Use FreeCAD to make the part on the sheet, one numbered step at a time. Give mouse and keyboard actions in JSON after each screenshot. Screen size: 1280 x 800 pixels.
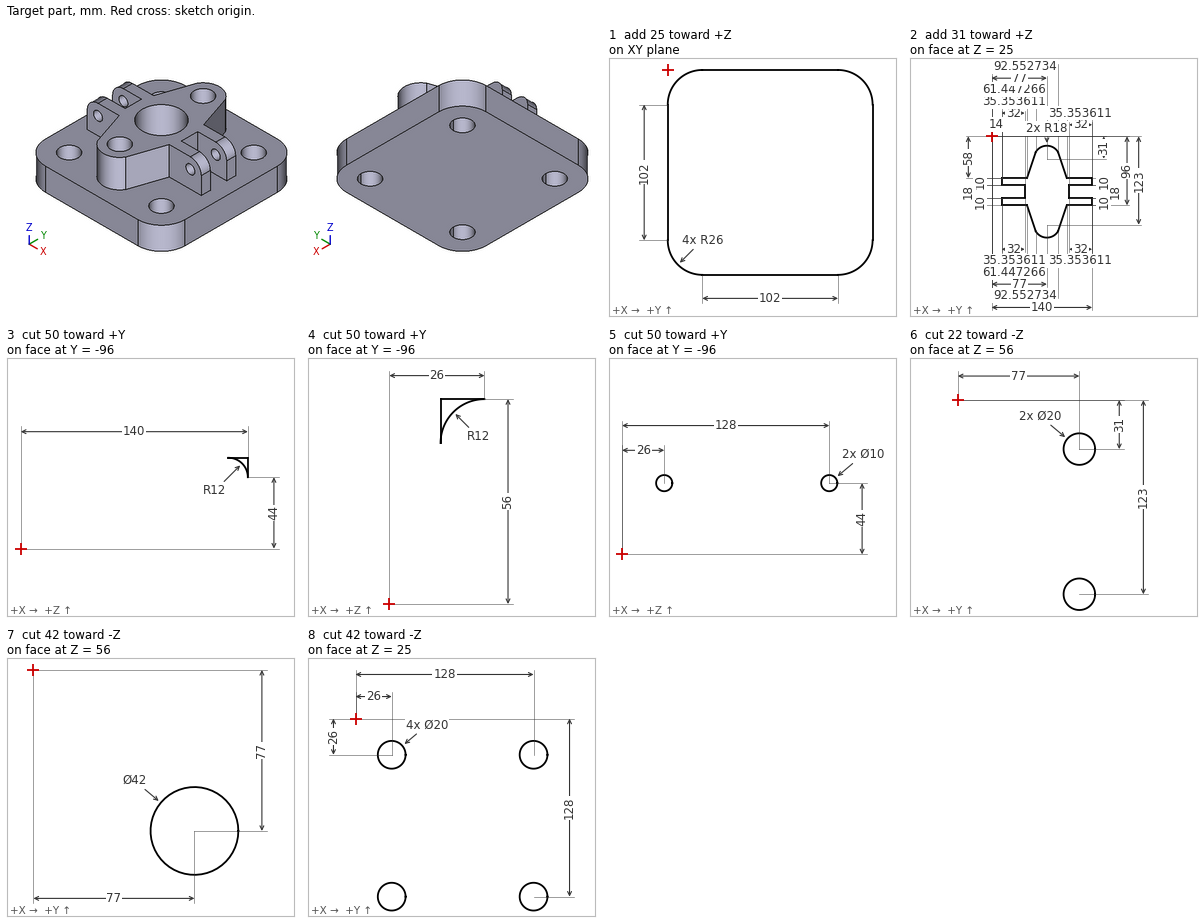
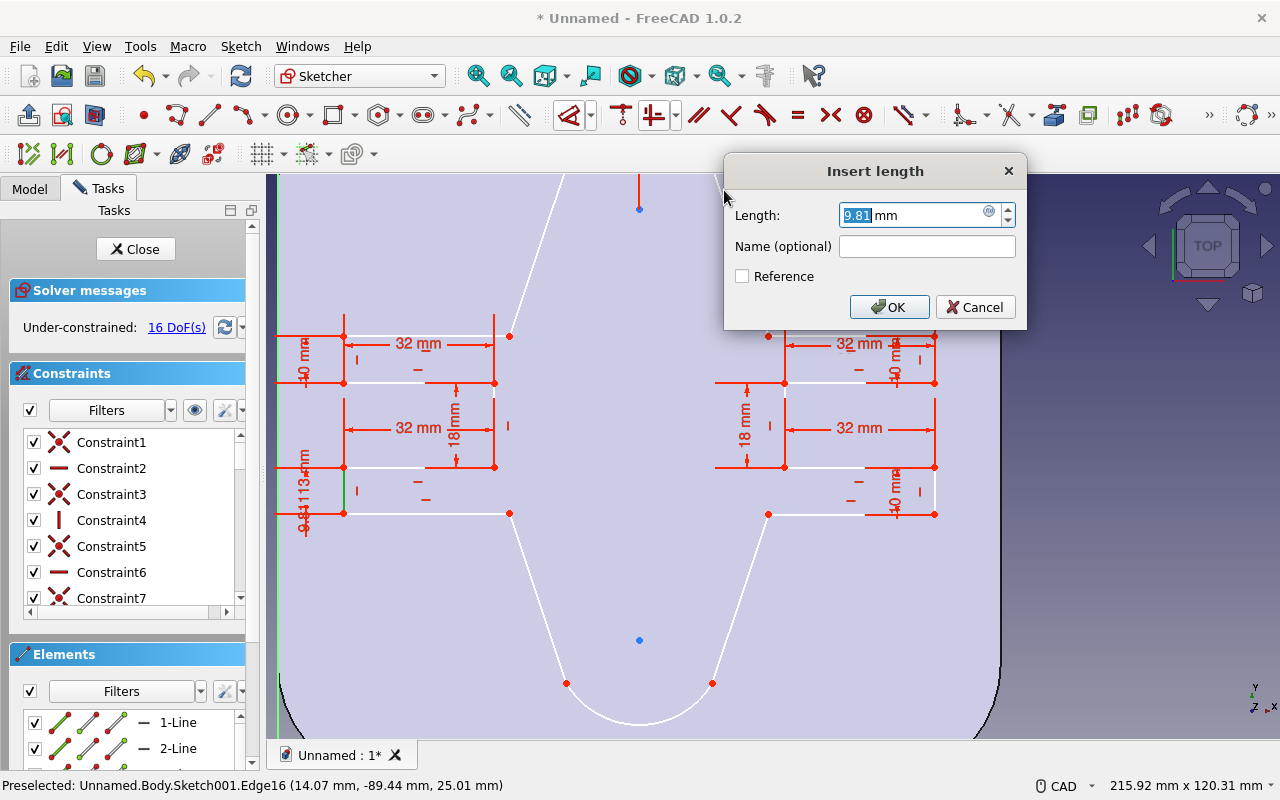
{"action": "type", "text": "10"}
{"action": "key", "text": "Return"}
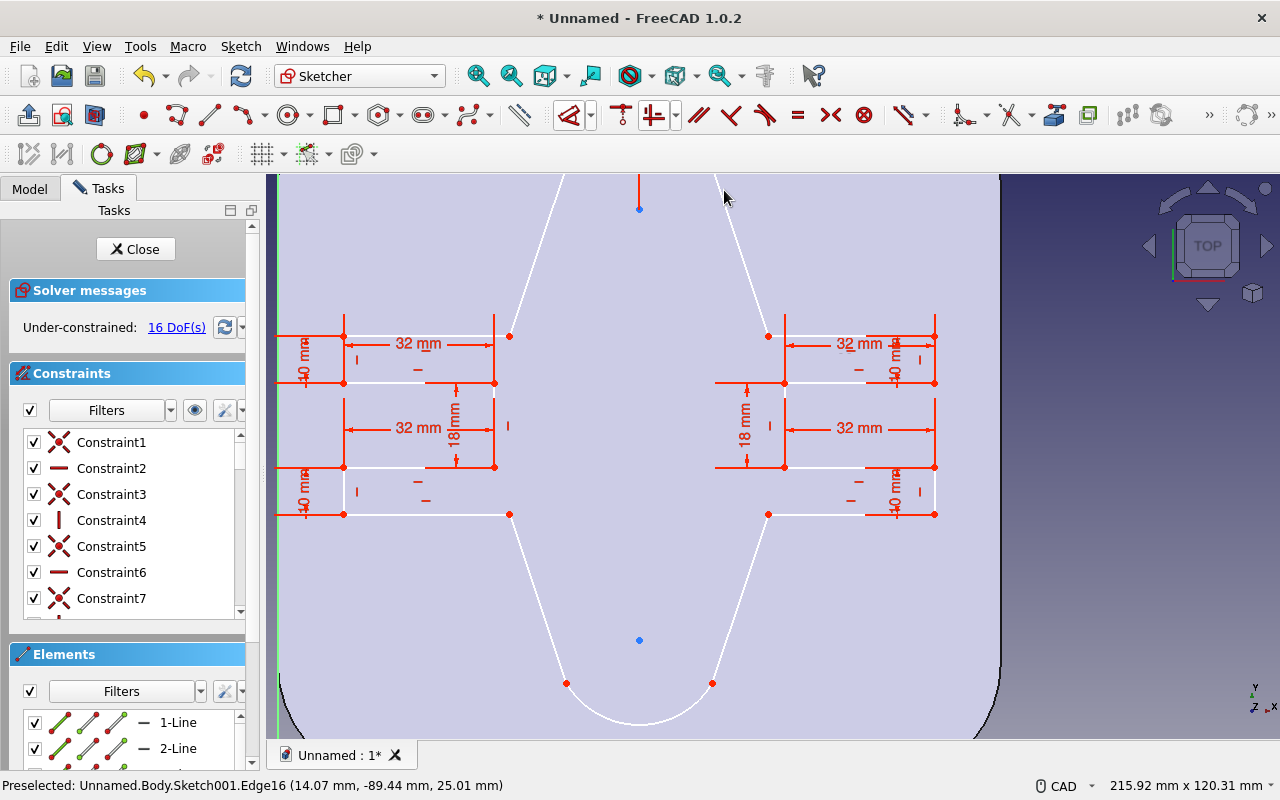
{"action": "left_click", "coordinate": [769, 515]}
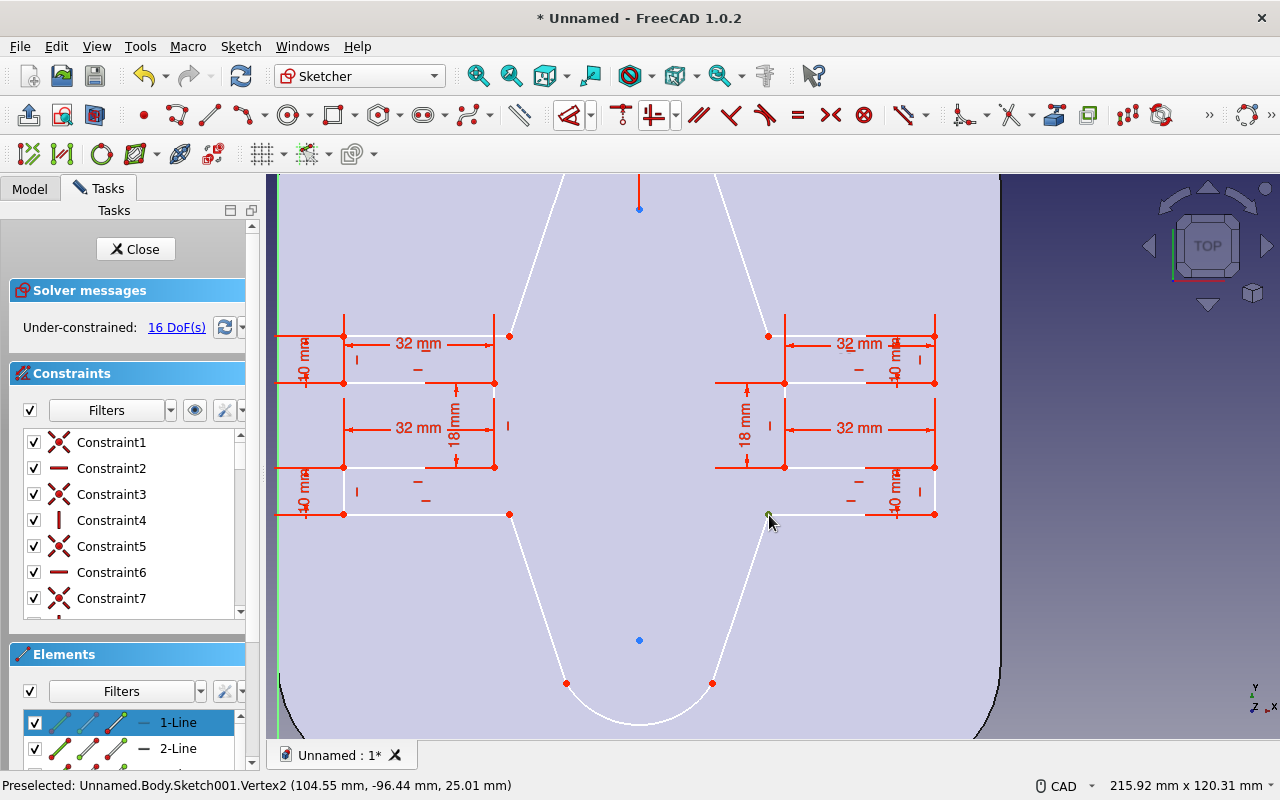
{"action": "key", "text": "i"}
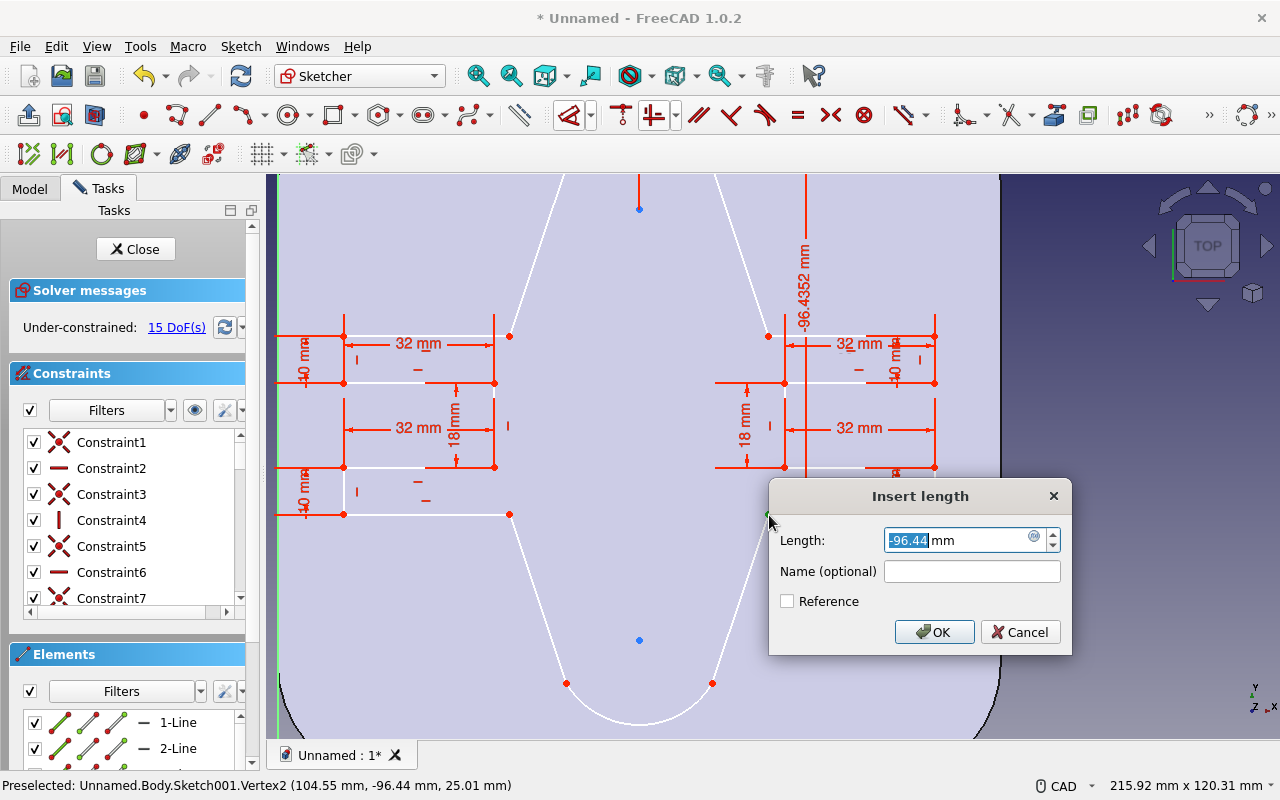
{"action": "type", "text": "-96"}
{"action": "key", "text": "Return"}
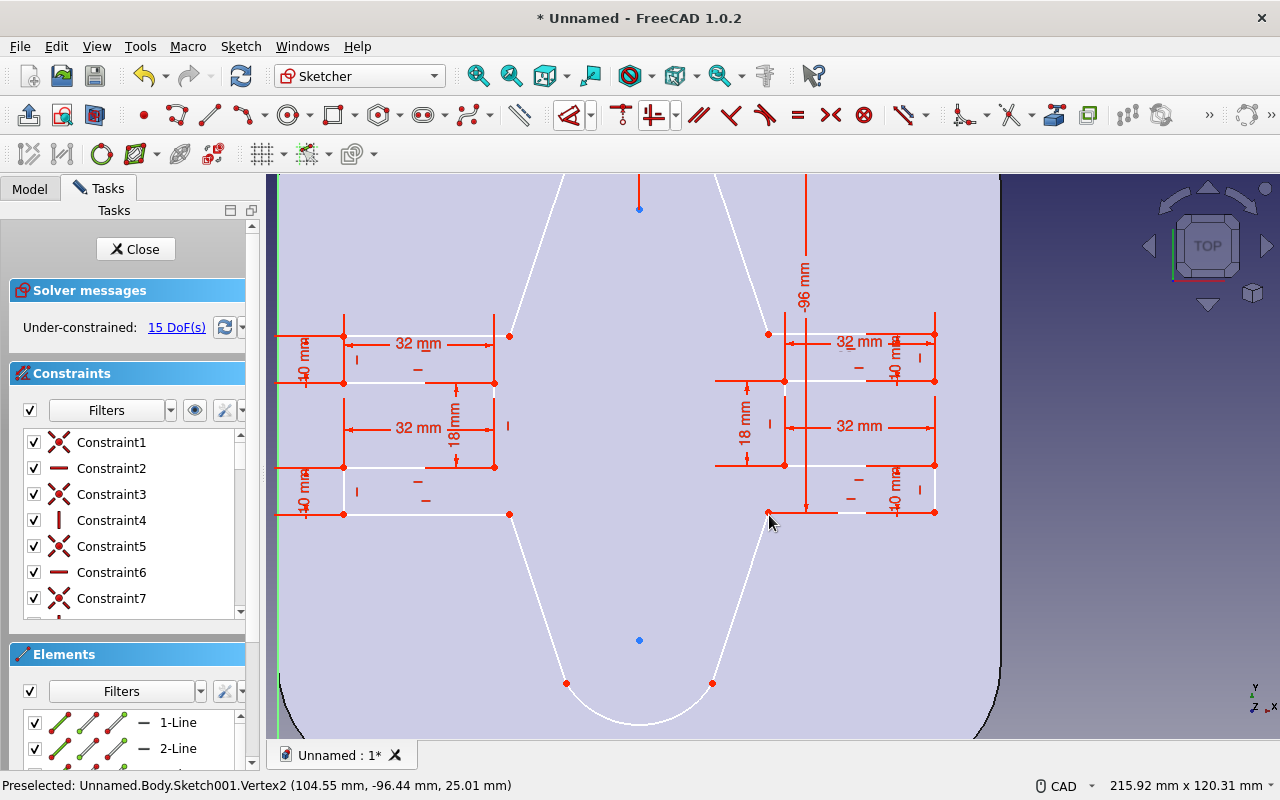
{"action": "left_click", "coordinate": [510, 336]}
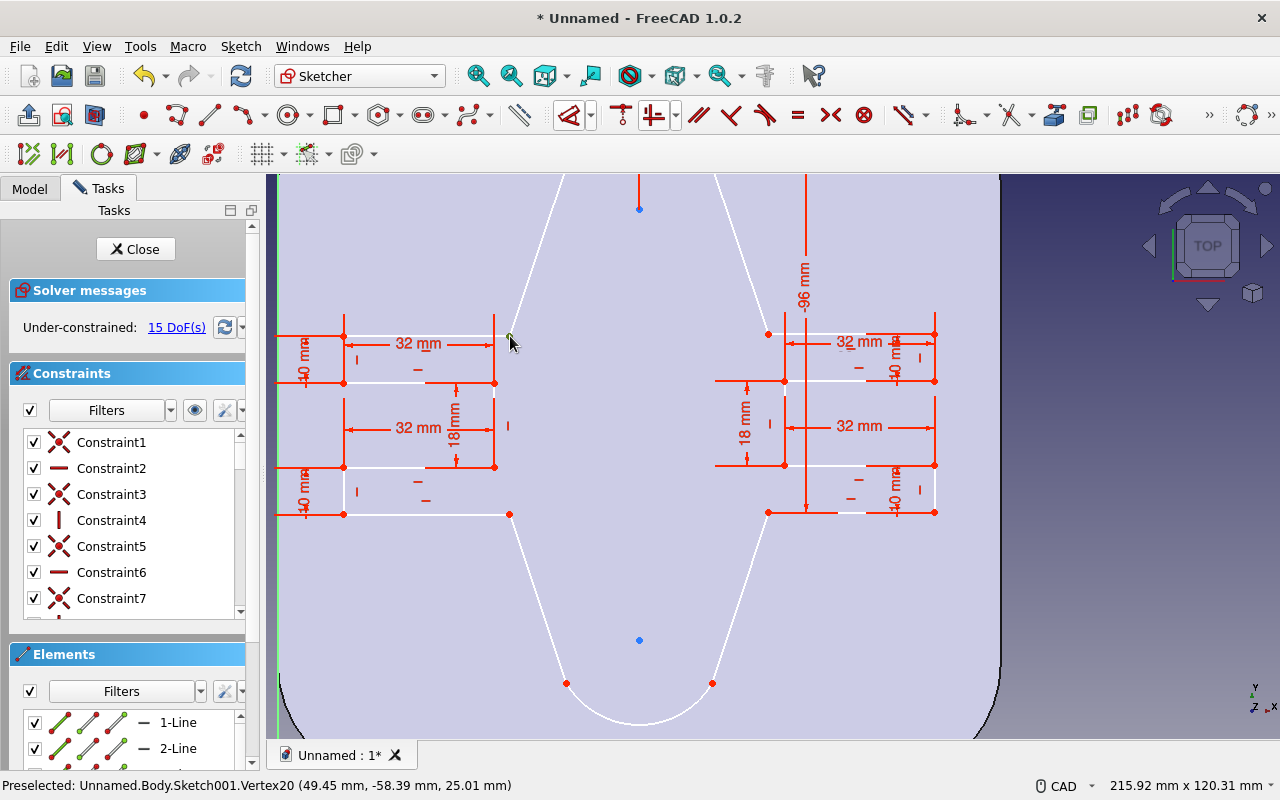
{"action": "key", "text": "i"}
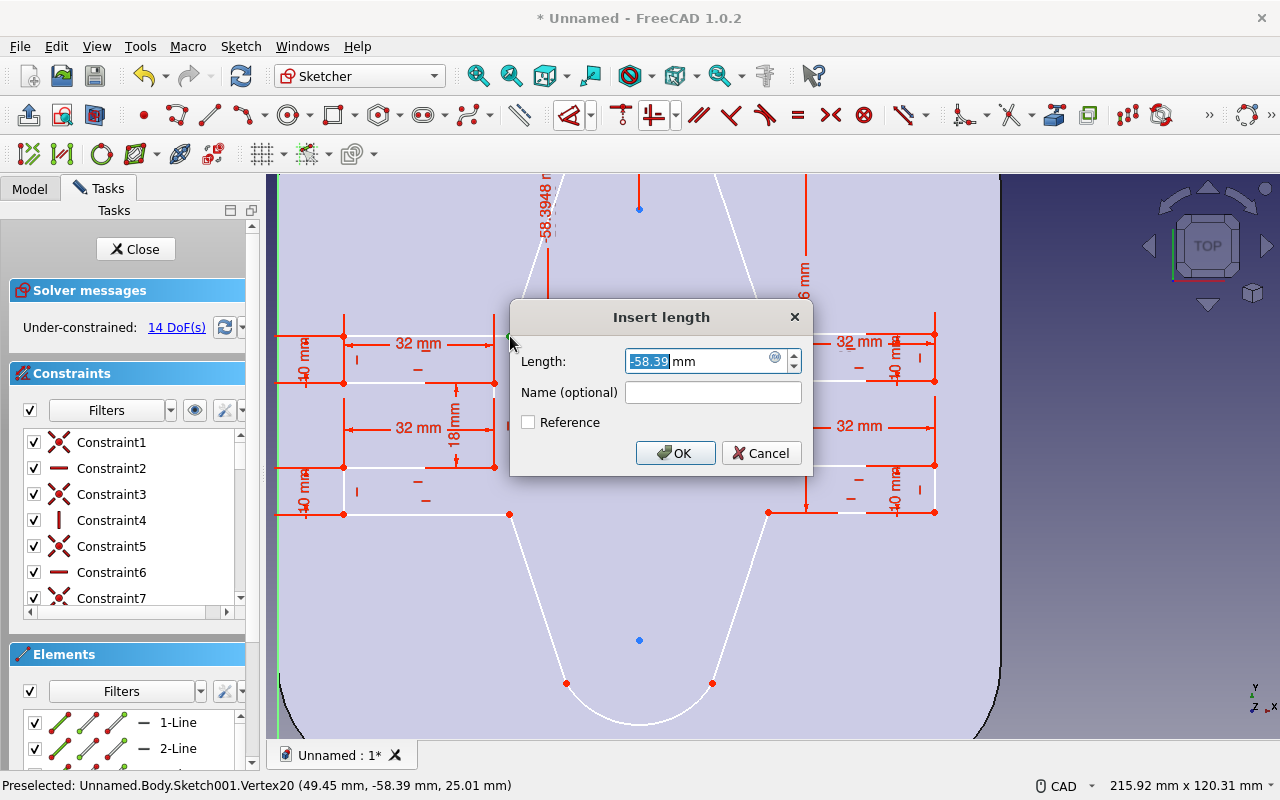
{"action": "type", "text": "-58"}
{"action": "key", "text": "Return"}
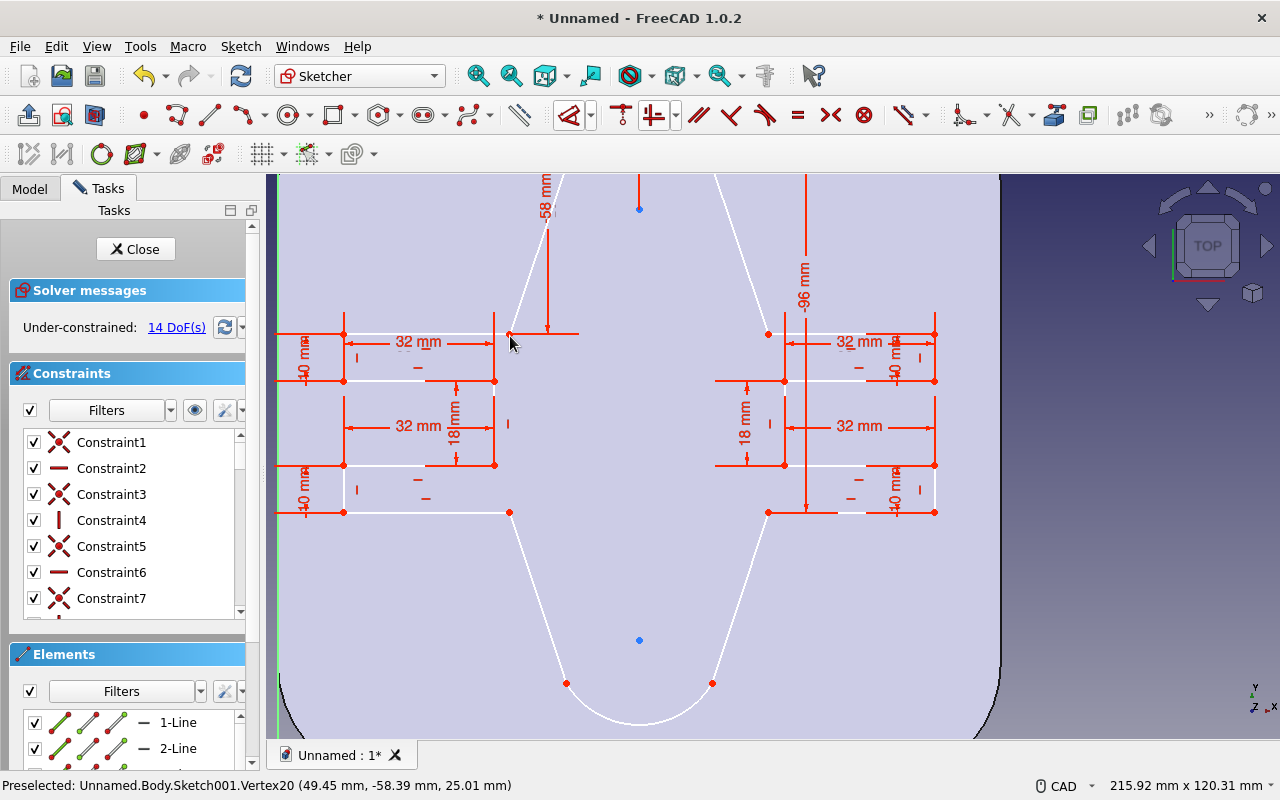
{"action": "left_click", "coordinate": [344, 334]}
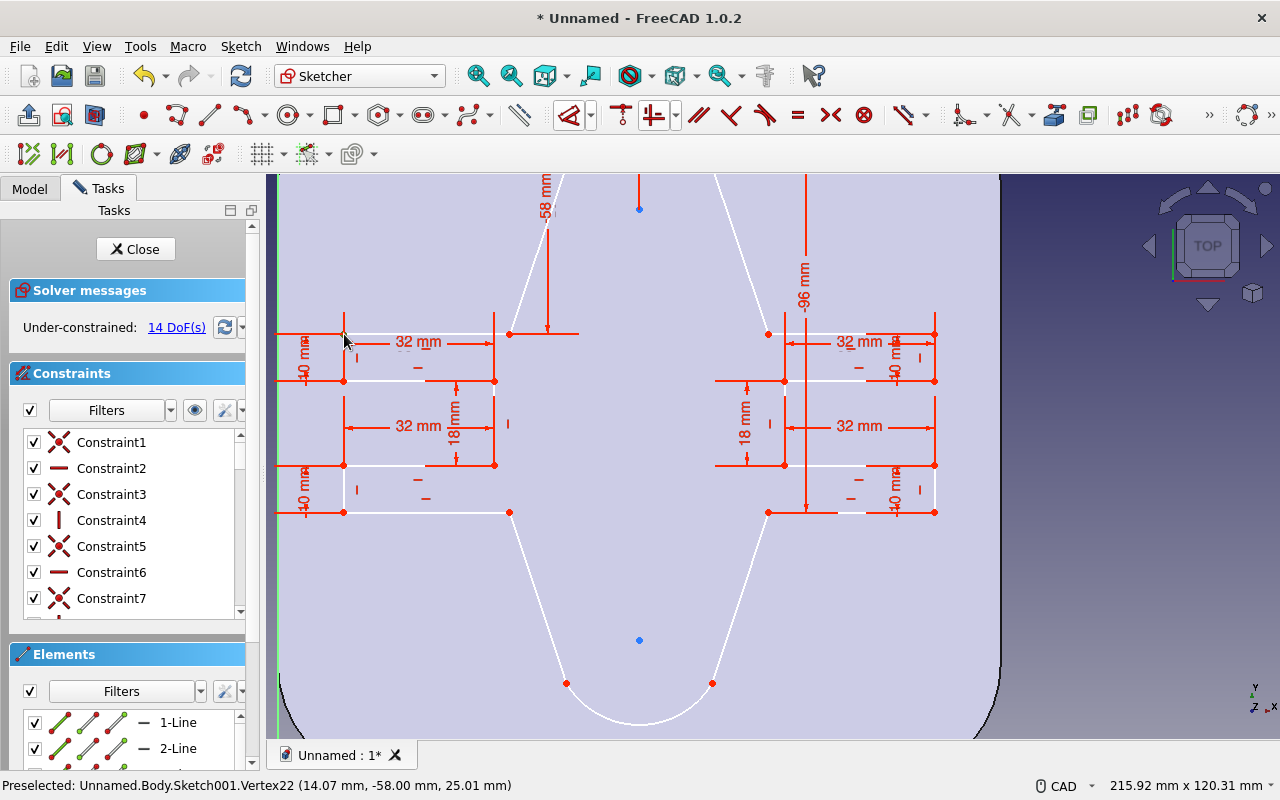
{"action": "key", "text": "l"}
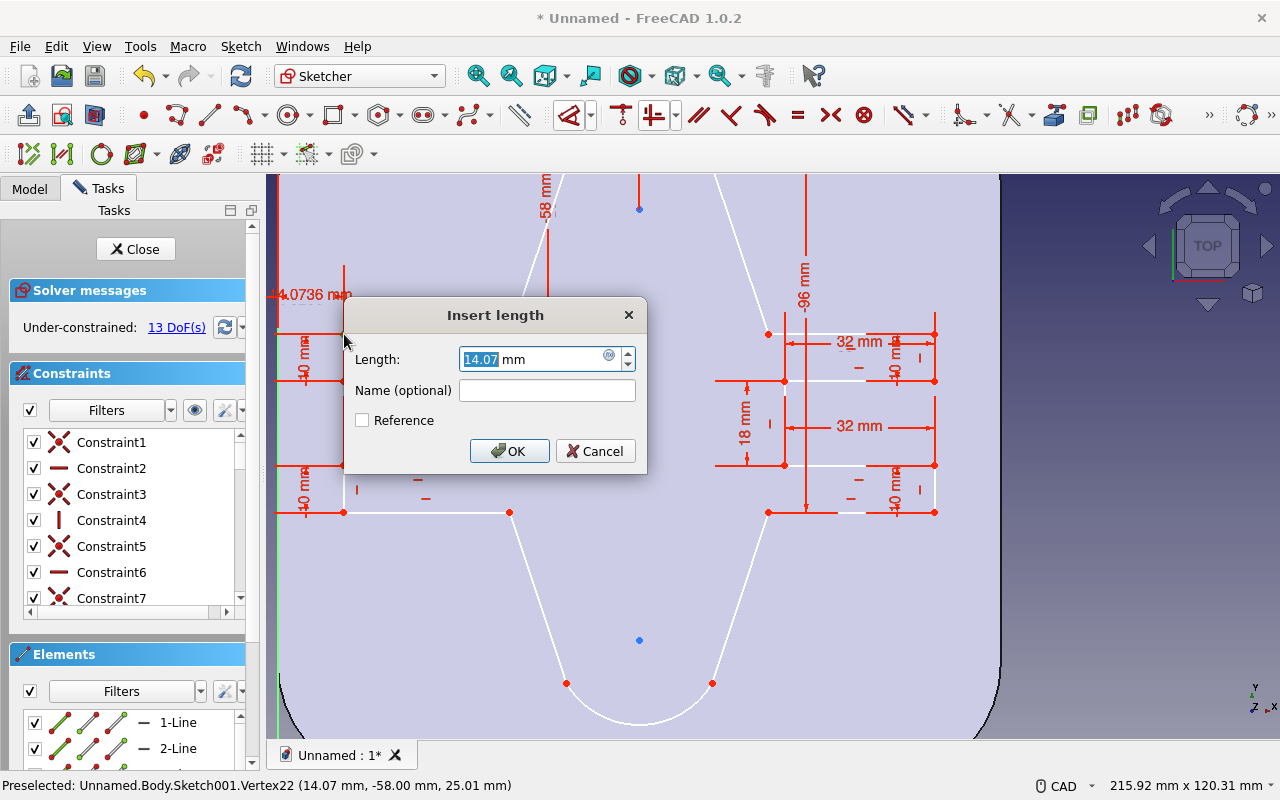
{"action": "type", "text": "14"}
{"action": "key", "text": "Return"}